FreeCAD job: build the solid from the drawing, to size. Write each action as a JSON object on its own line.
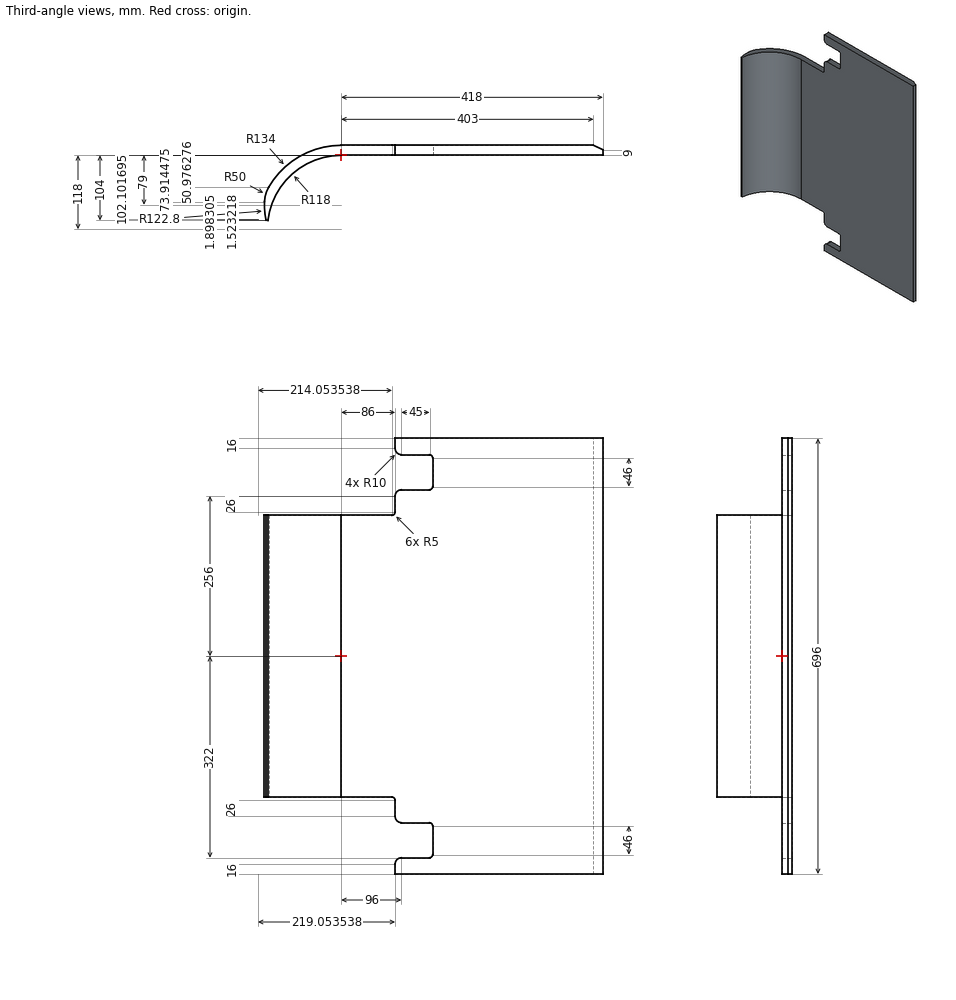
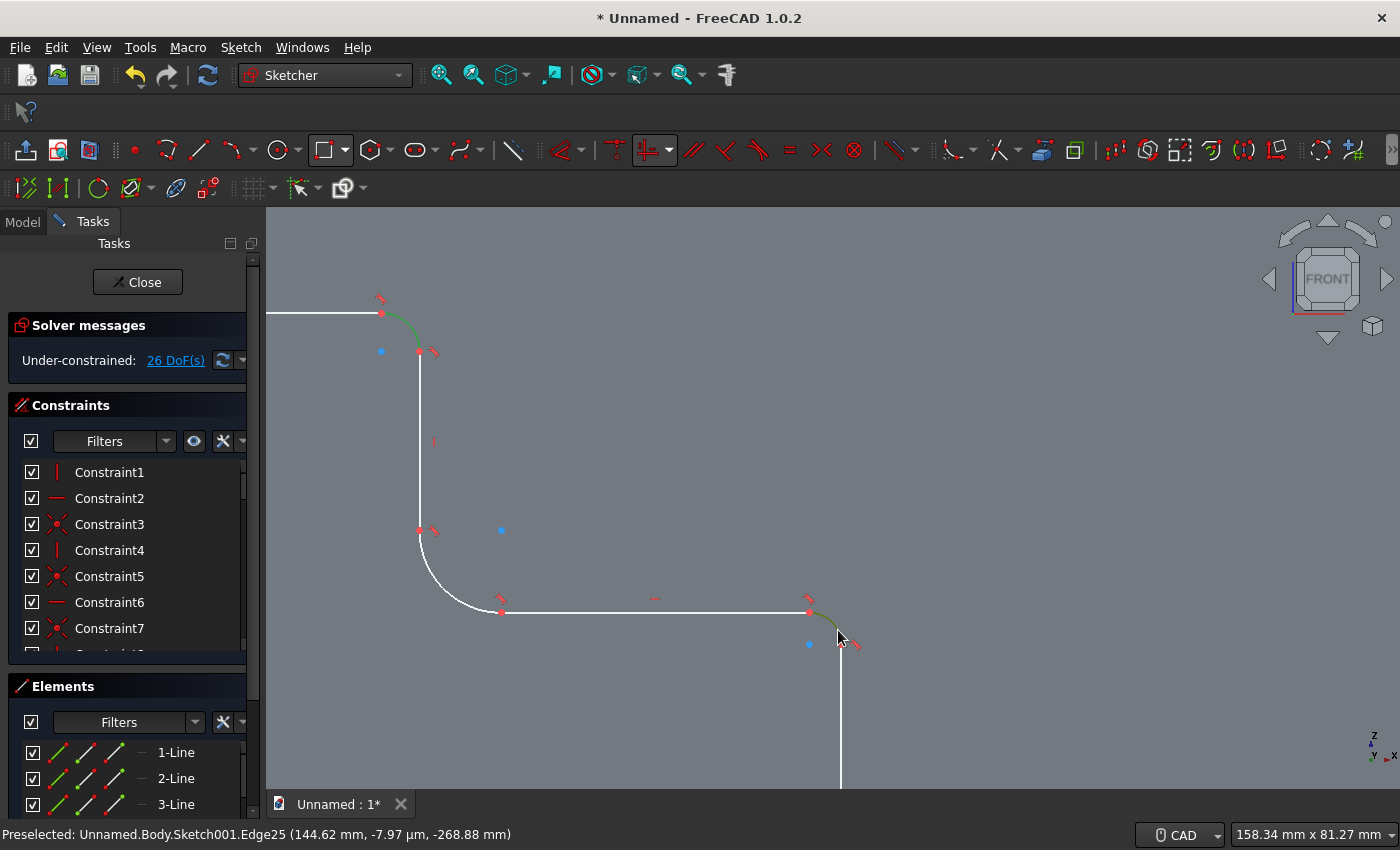
{"action": "scroll", "coordinate": [838, 642], "scroll_direction": "down", "scroll_amount": 13}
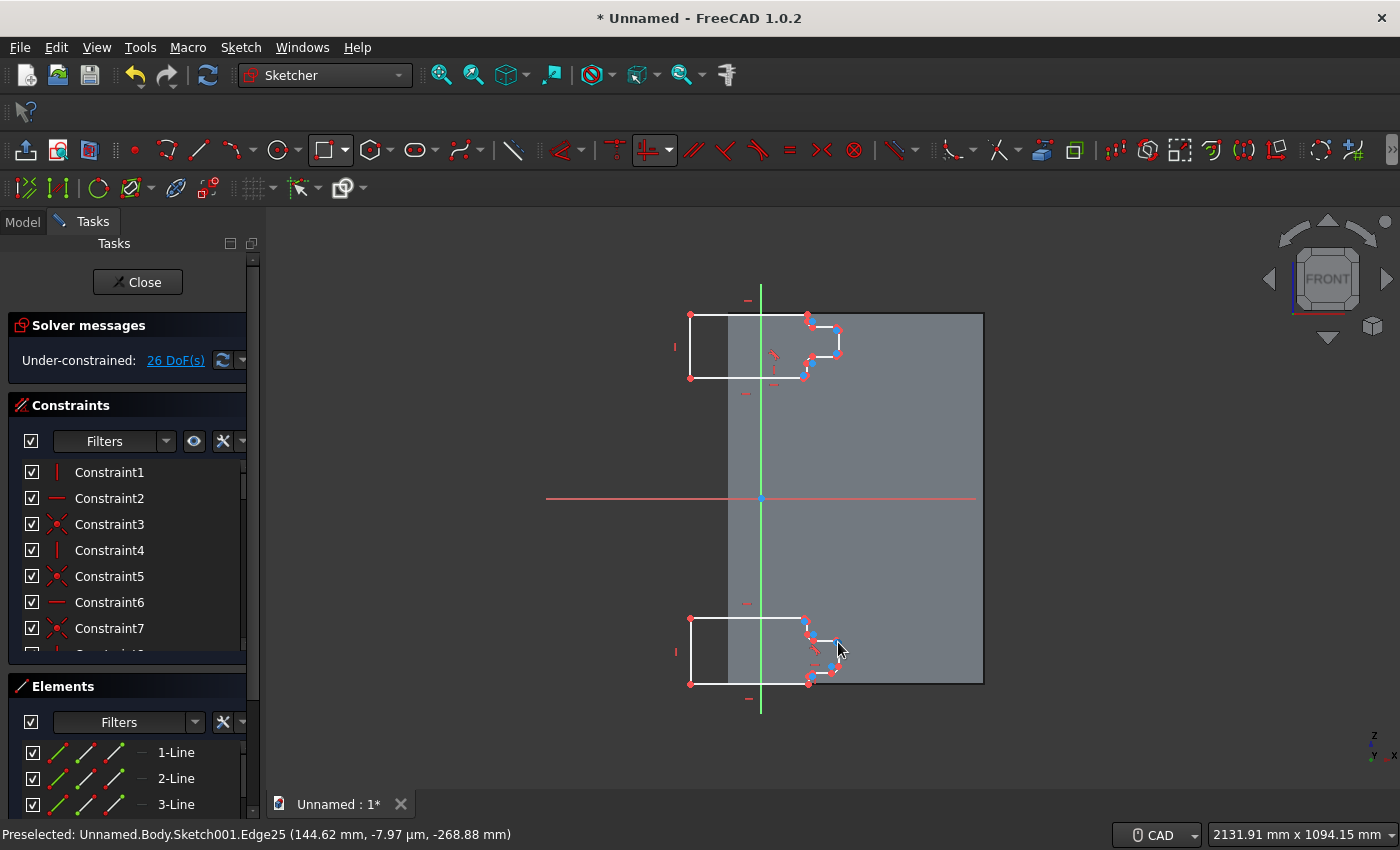
{"action": "scroll", "coordinate": [835, 672], "scroll_direction": "up", "scroll_amount": 8}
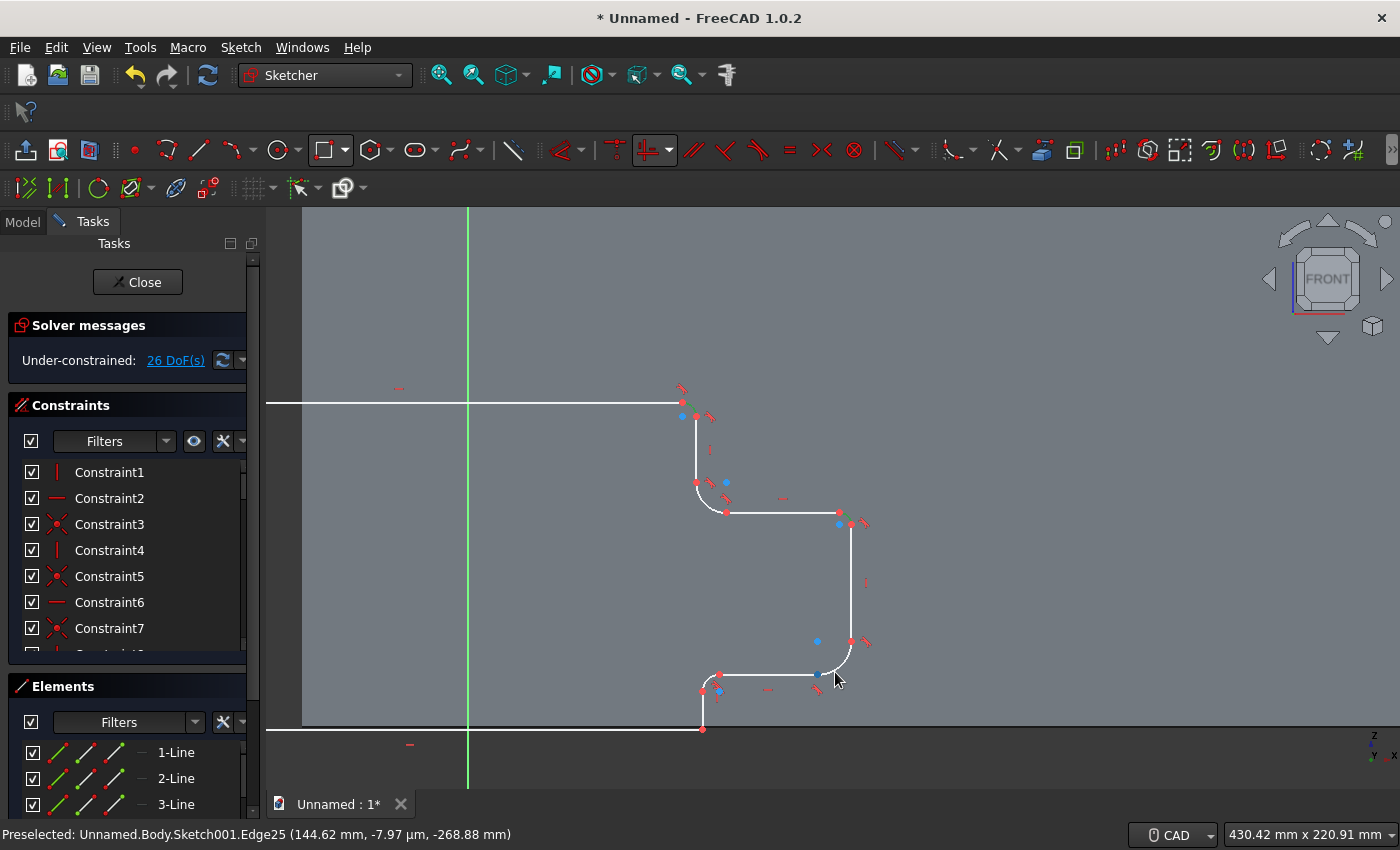
{"action": "left_click", "coordinate": [833, 671]}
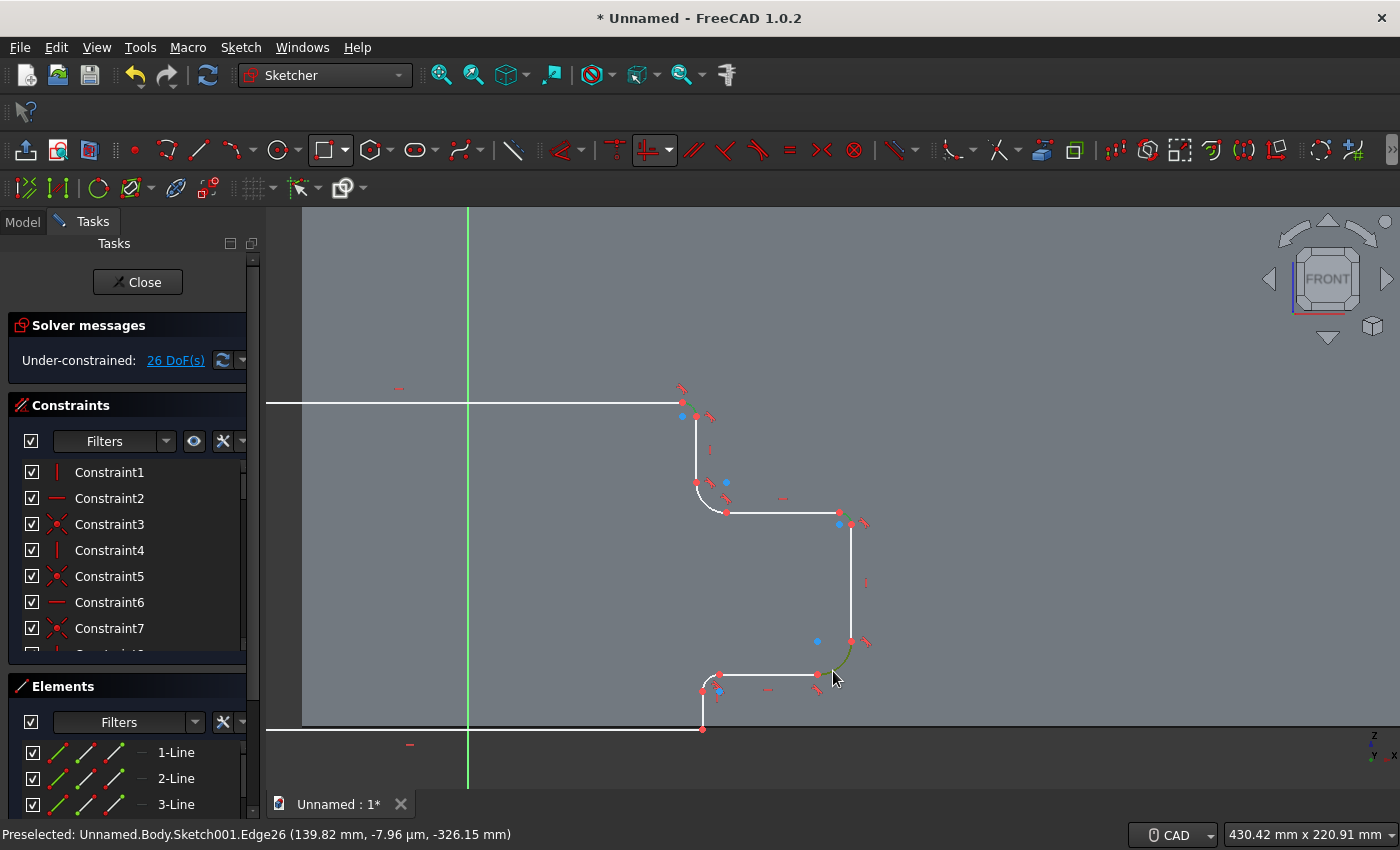
{"action": "left_click", "coordinate": [790, 150]}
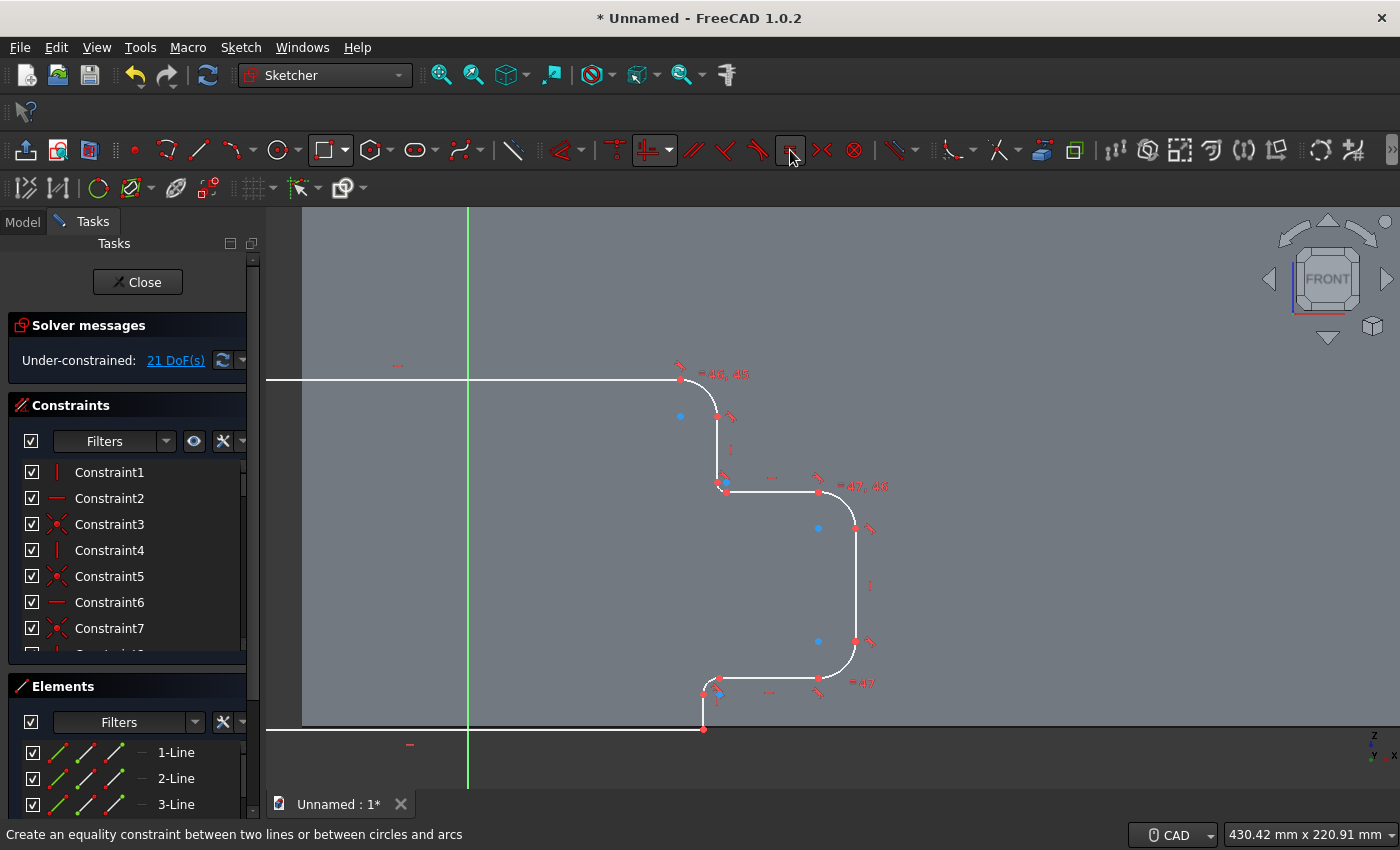
{"action": "scroll", "coordinate": [835, 672], "scroll_direction": "down", "scroll_amount": 8}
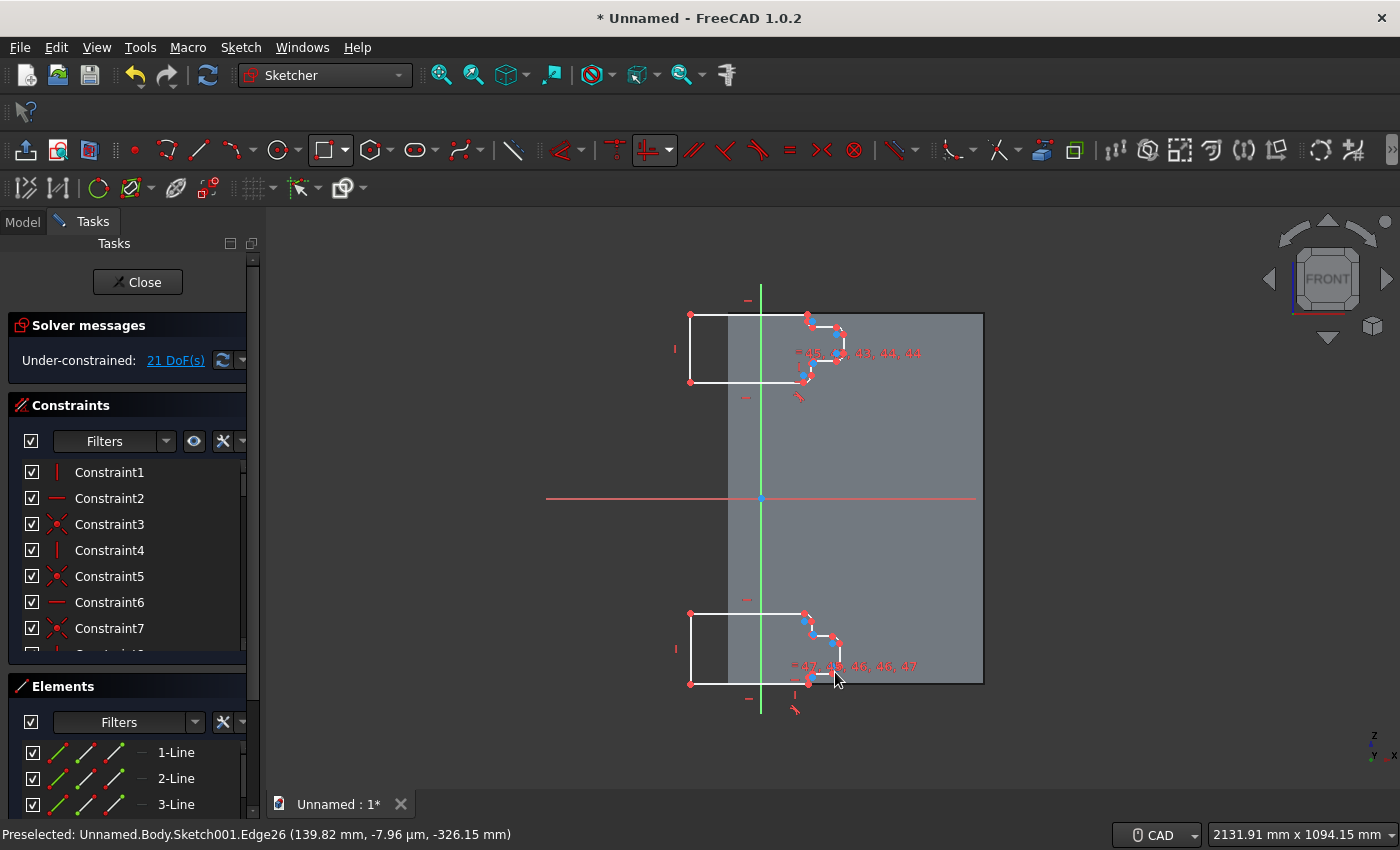
{"action": "scroll", "coordinate": [808, 324], "scroll_direction": "up", "scroll_amount": 9}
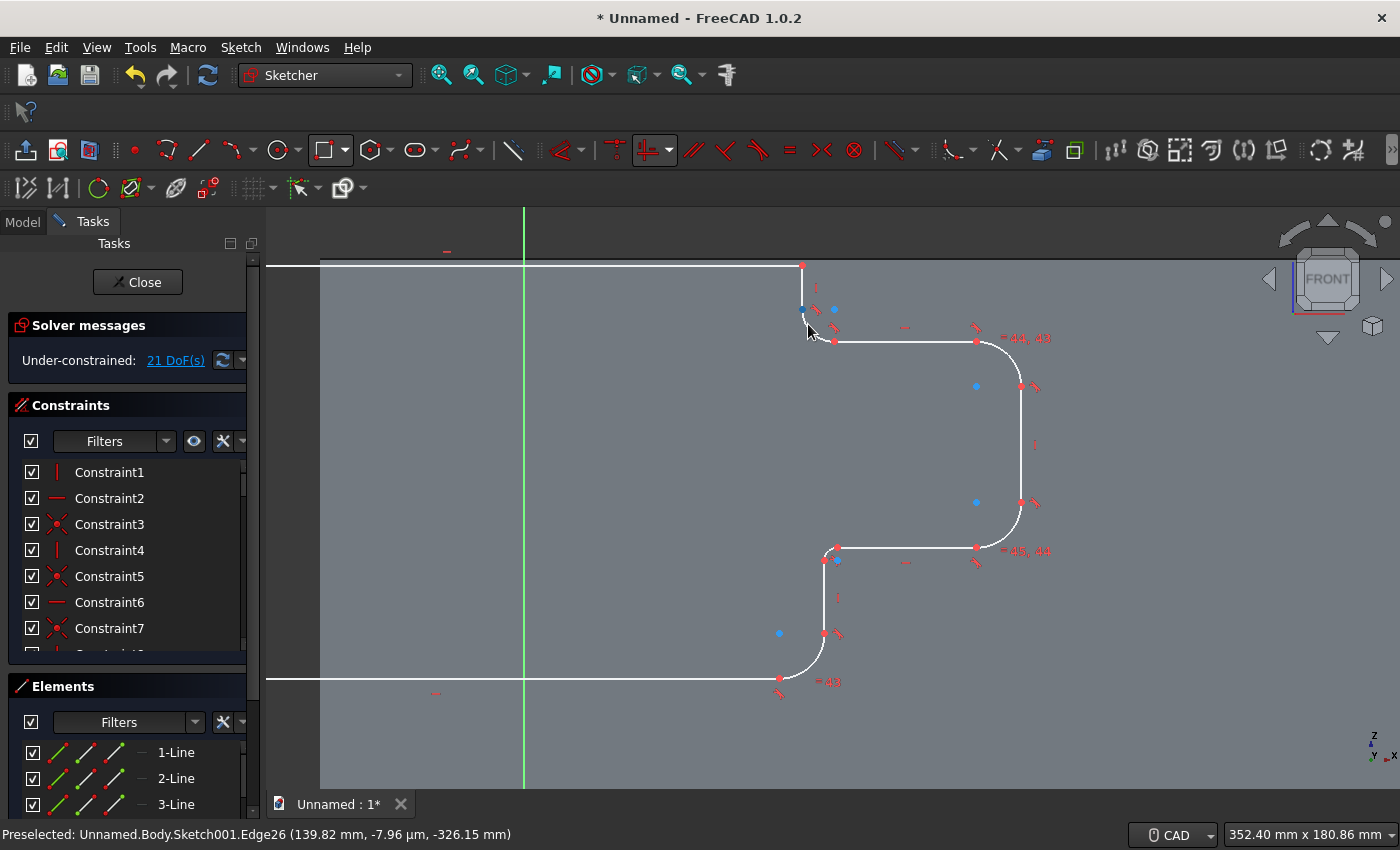
{"action": "left_click", "coordinate": [806, 324]}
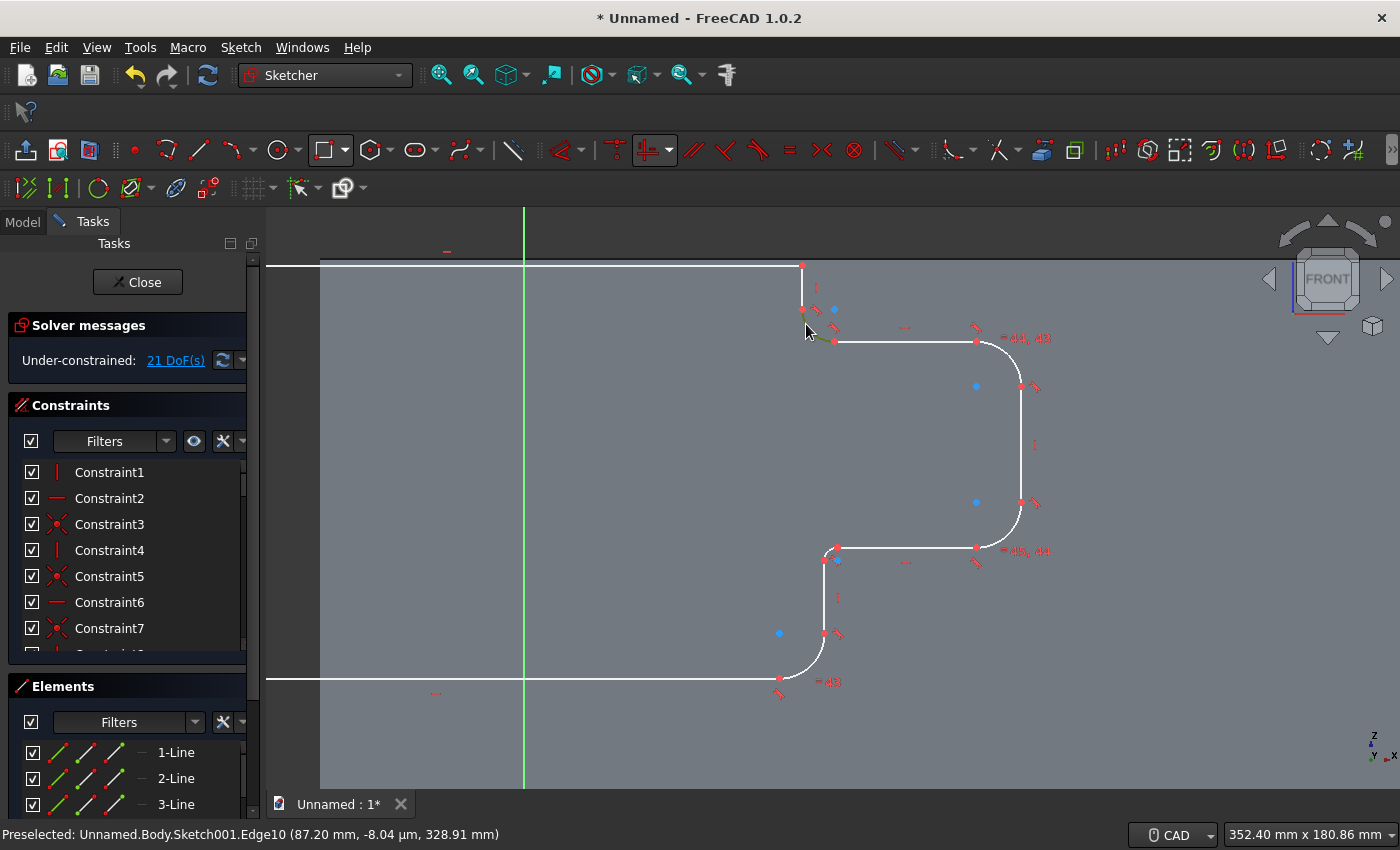
{"action": "scroll", "coordinate": [828, 551], "scroll_direction": "up", "scroll_amount": 2}